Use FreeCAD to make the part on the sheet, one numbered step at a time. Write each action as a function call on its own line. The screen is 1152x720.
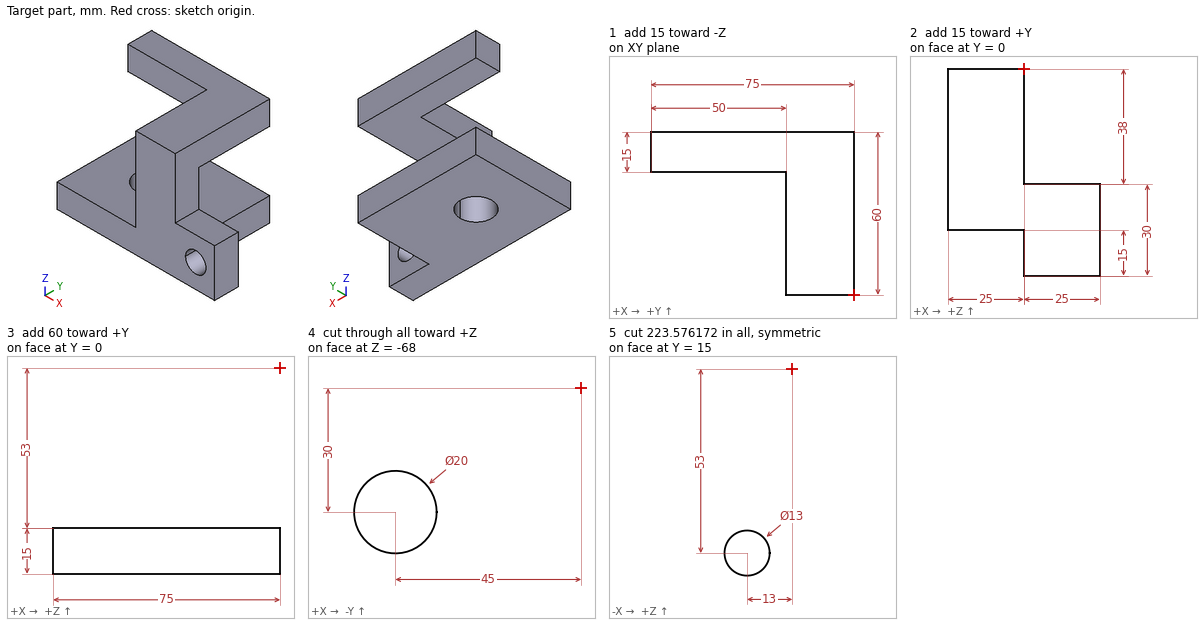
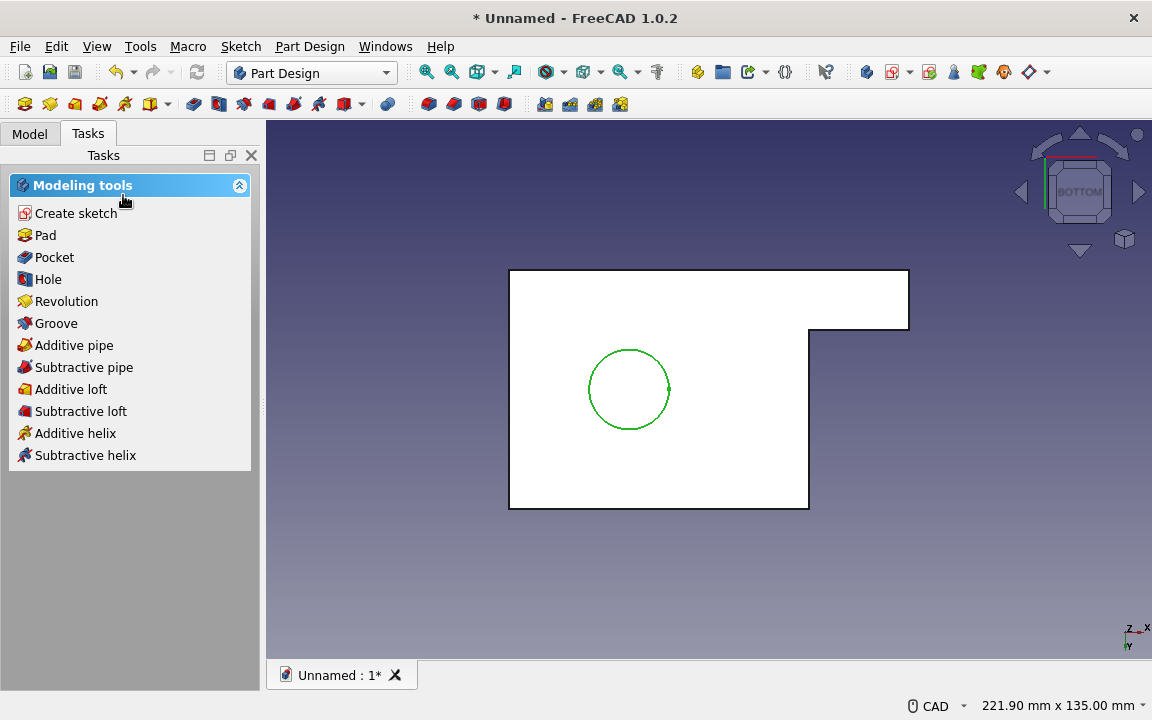
click(194, 104)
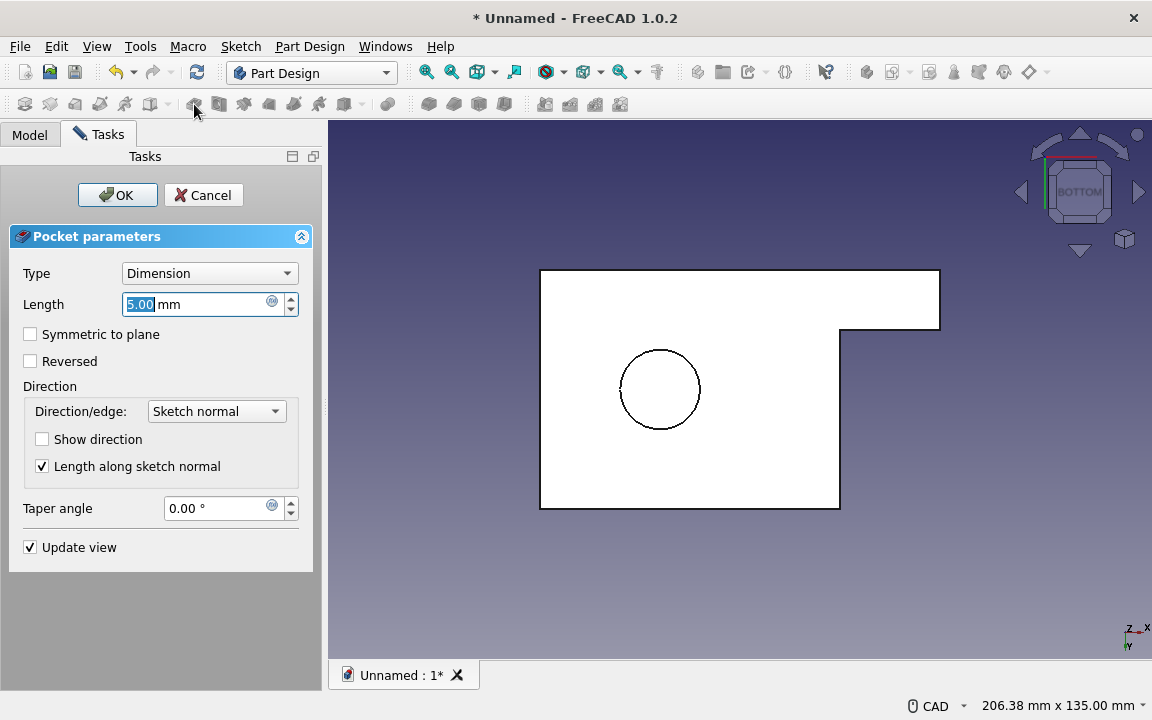
click(210, 274)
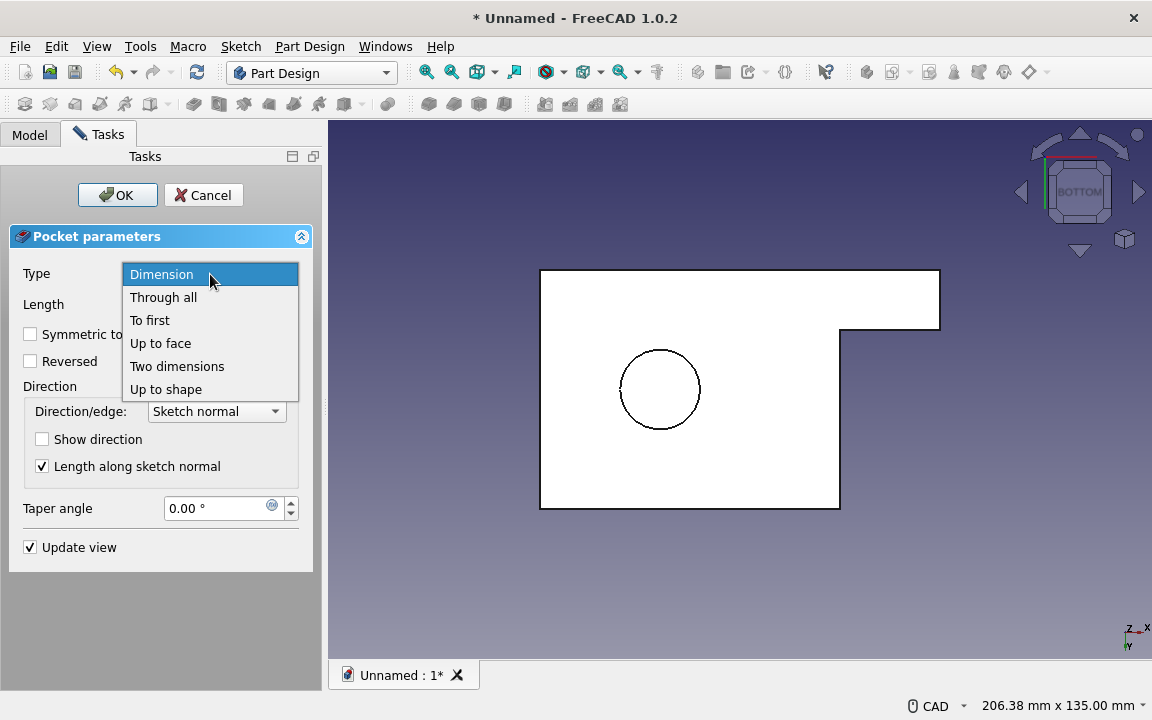
click(208, 298)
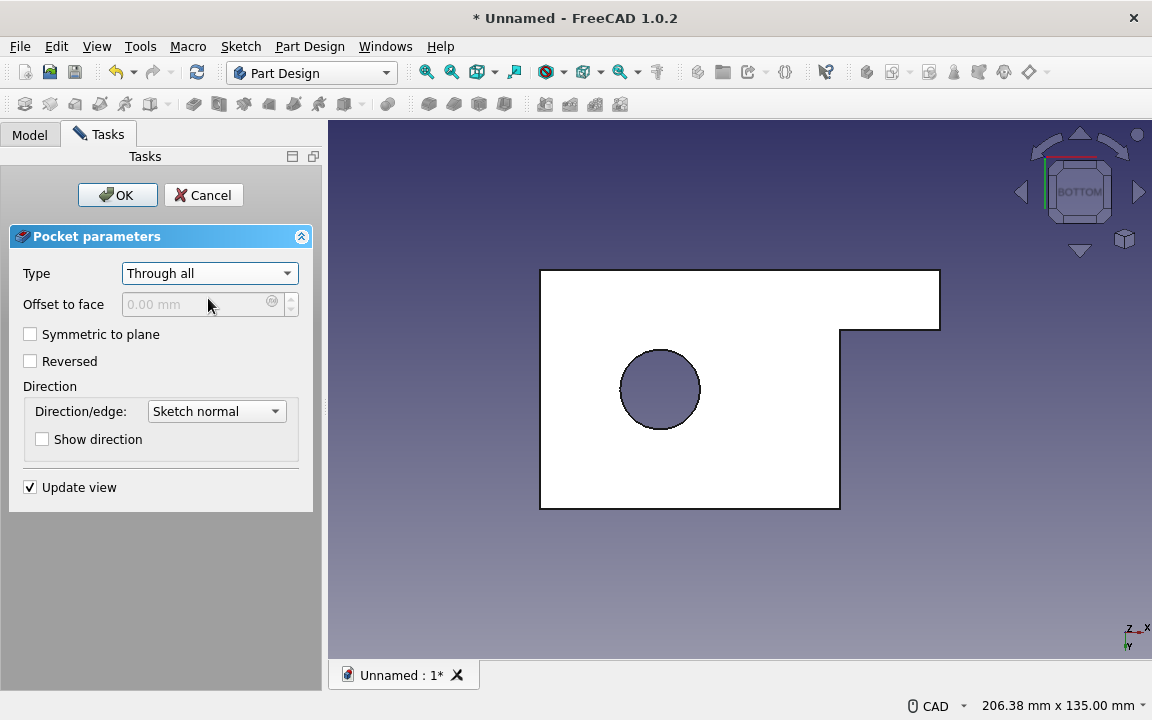
click(118, 195)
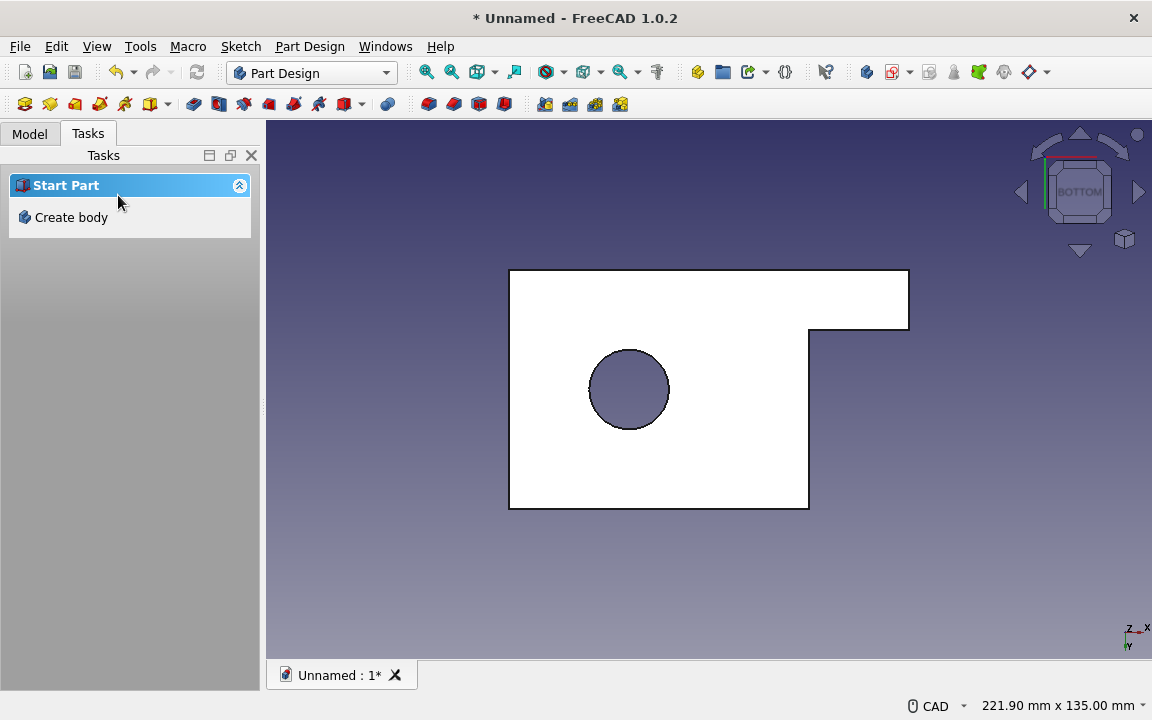
key(4)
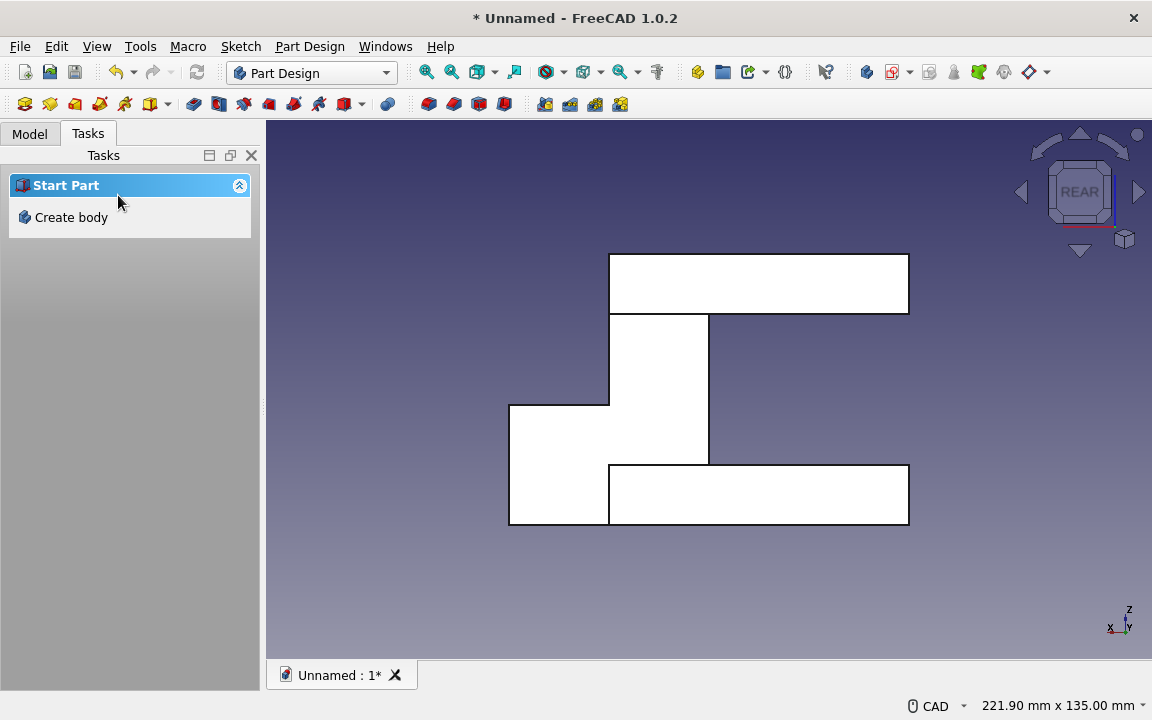
click(552, 449)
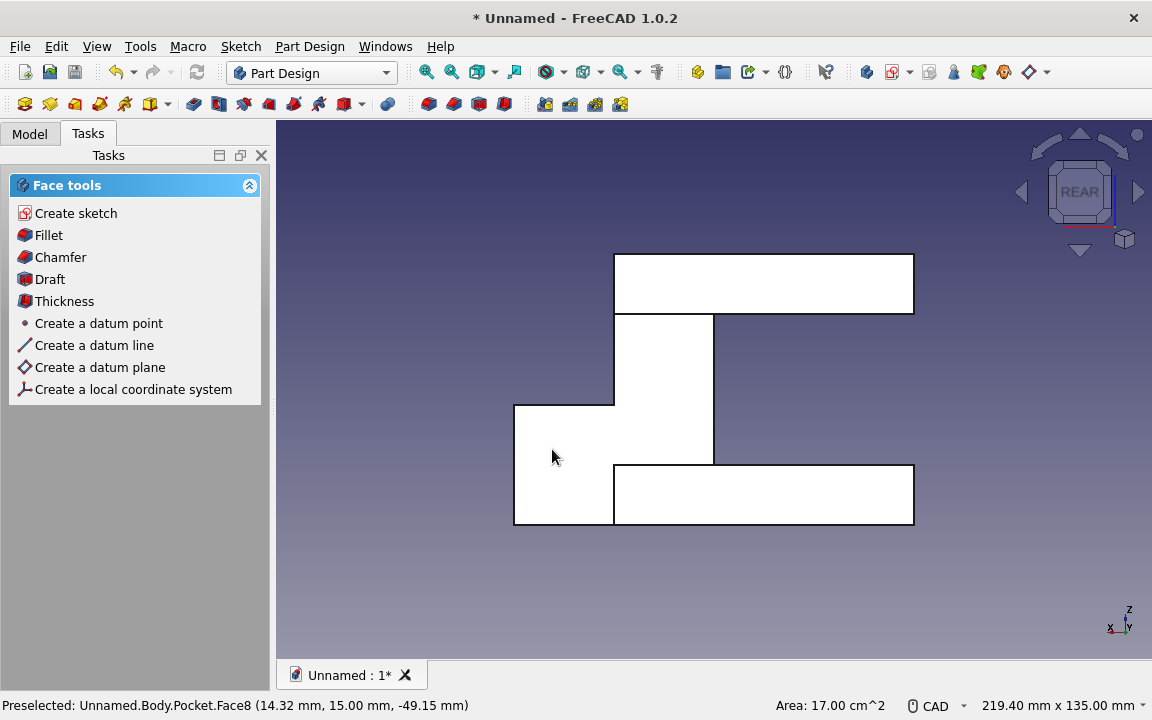
click(892, 72)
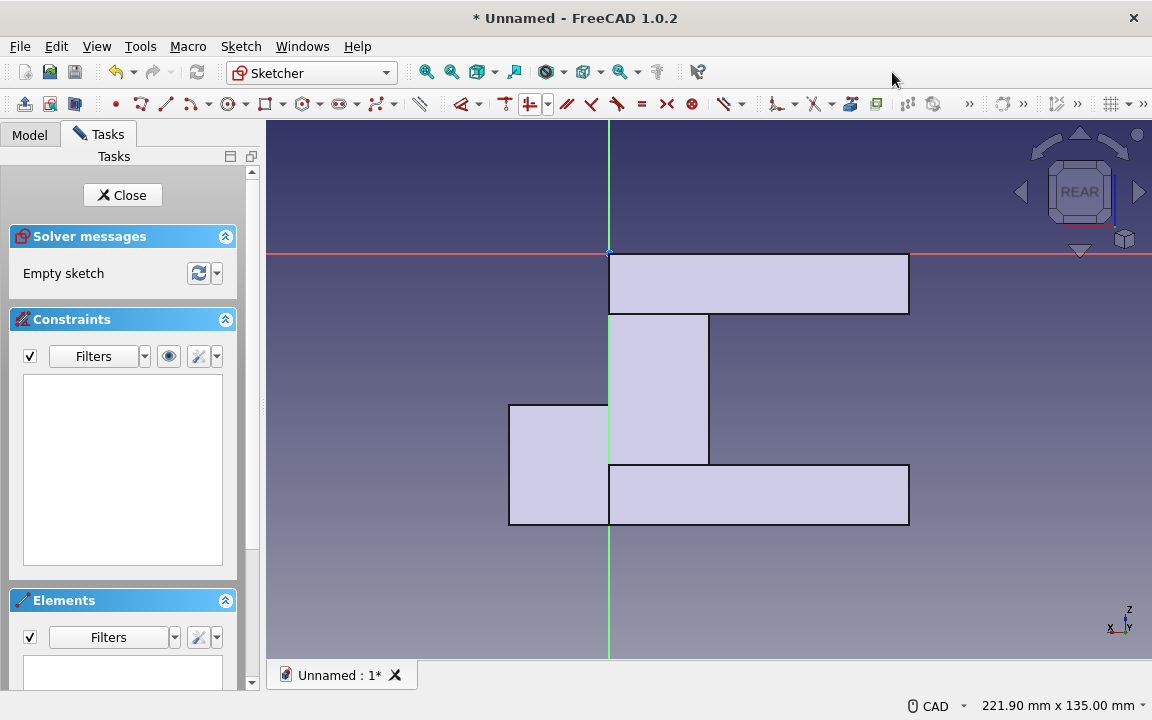
click(75, 104)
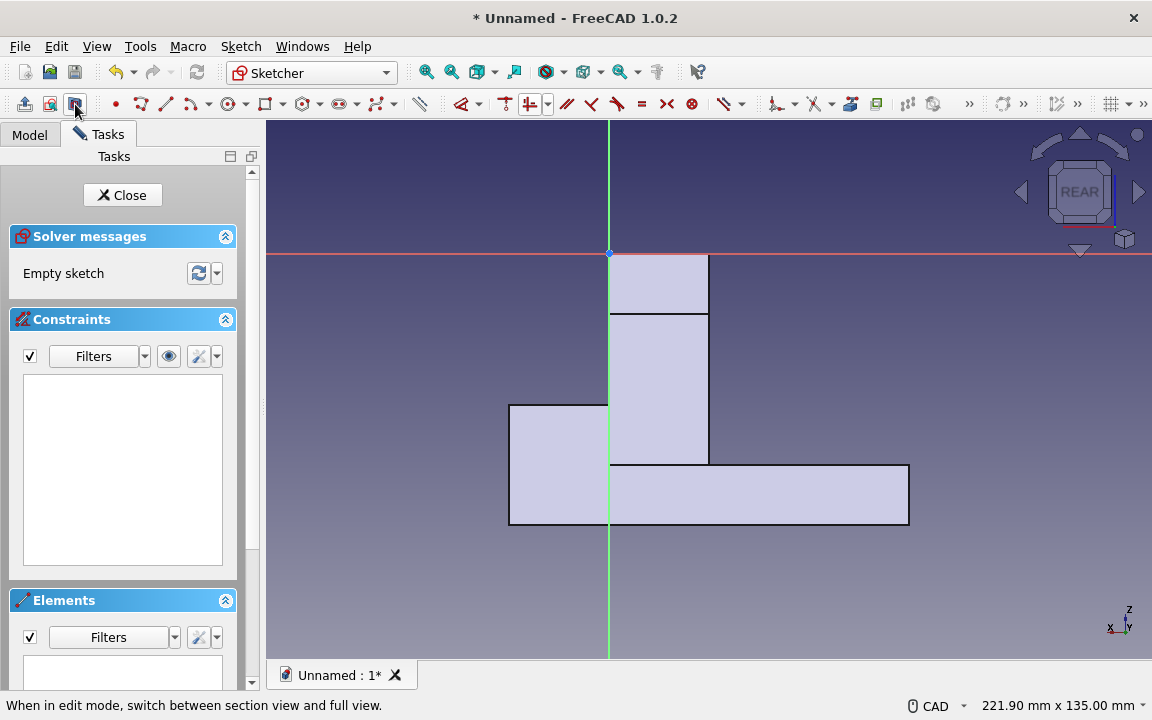
scroll(541, 480, up, 9)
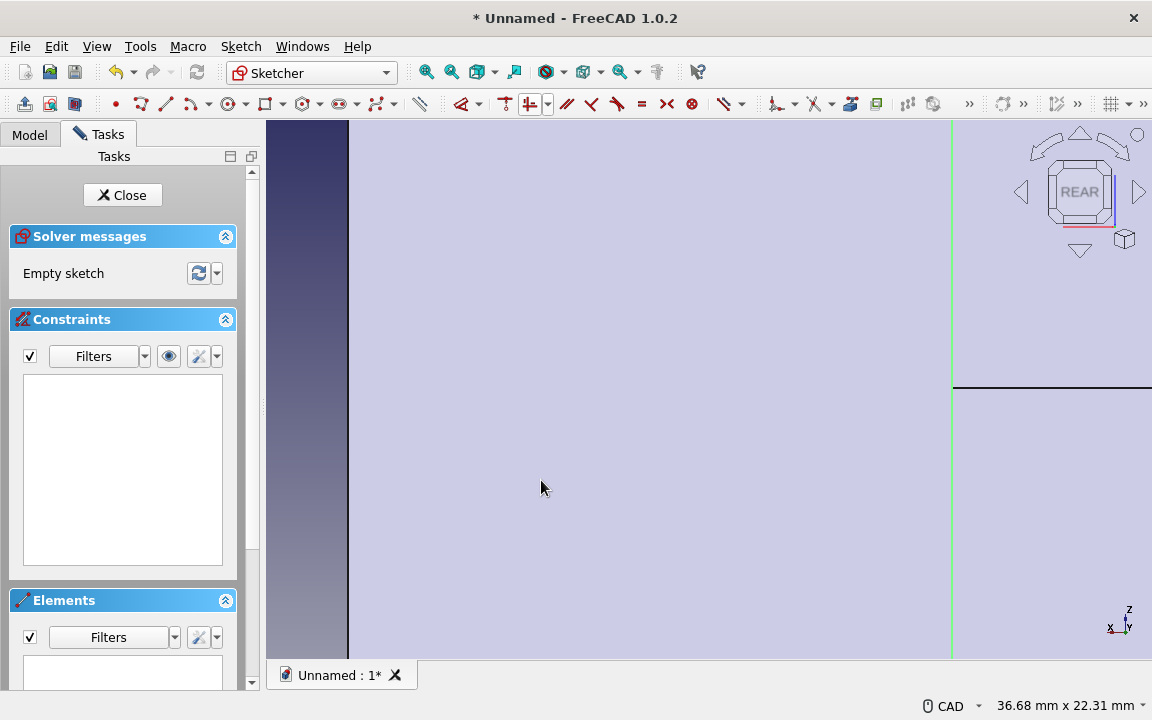
key(g)
key(c)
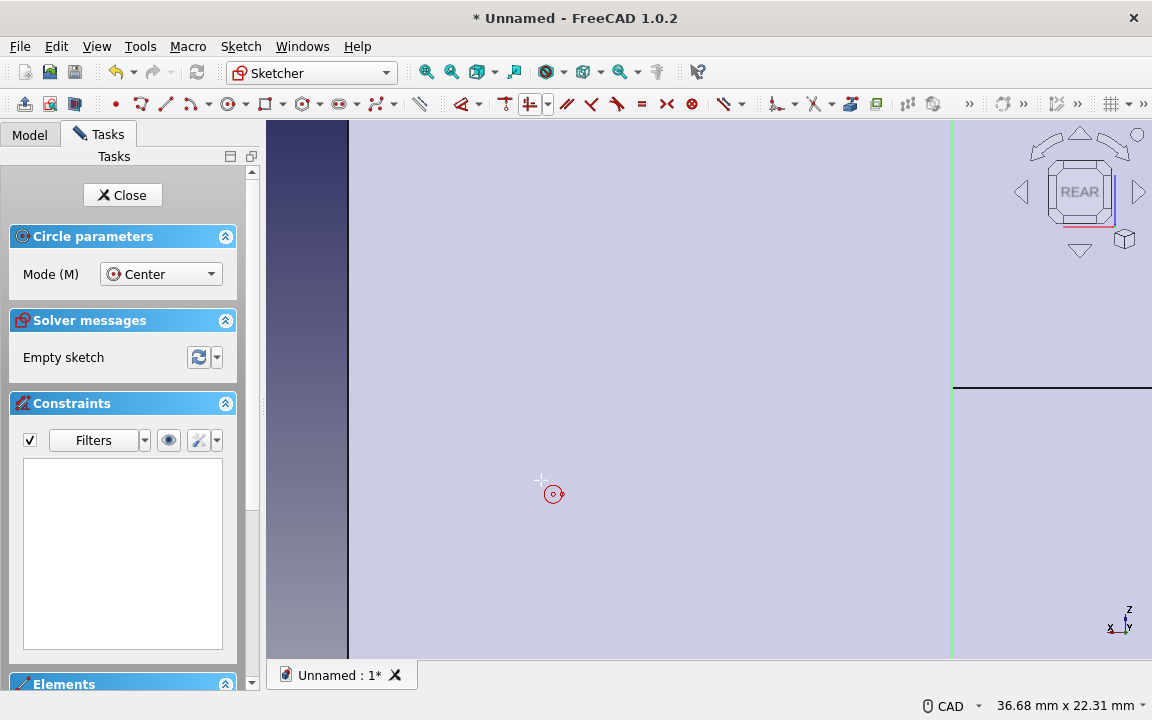
click(638, 388)
click(749, 277)
key(Escape)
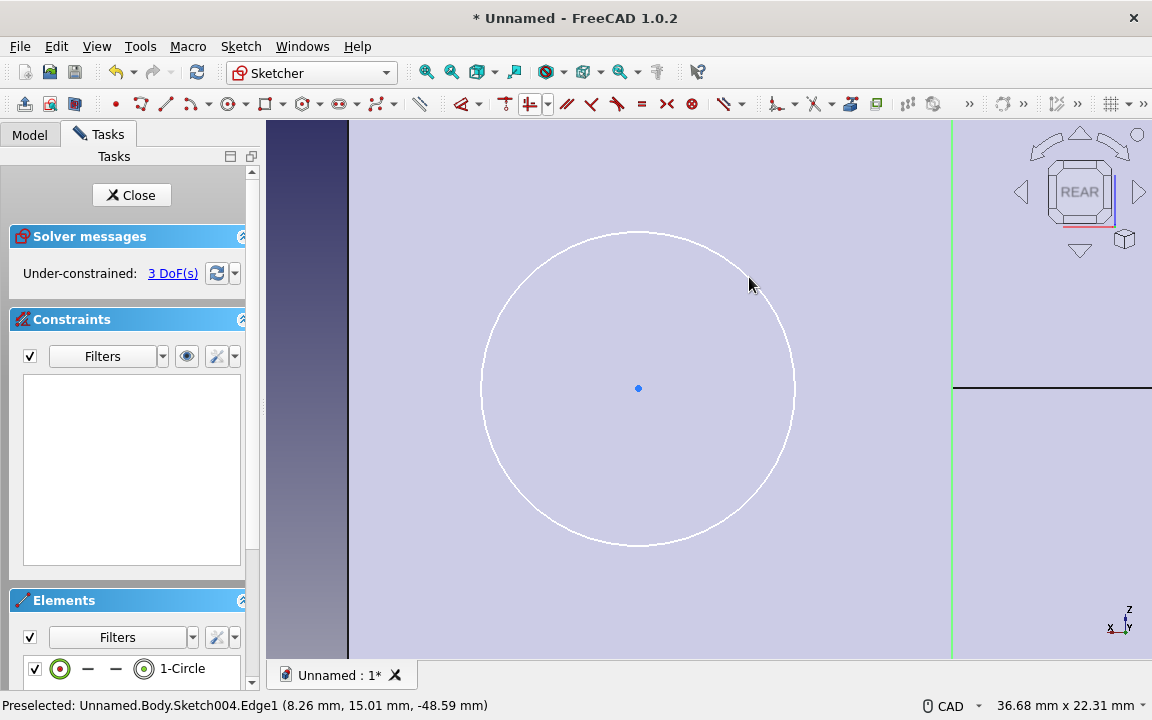
key(d)